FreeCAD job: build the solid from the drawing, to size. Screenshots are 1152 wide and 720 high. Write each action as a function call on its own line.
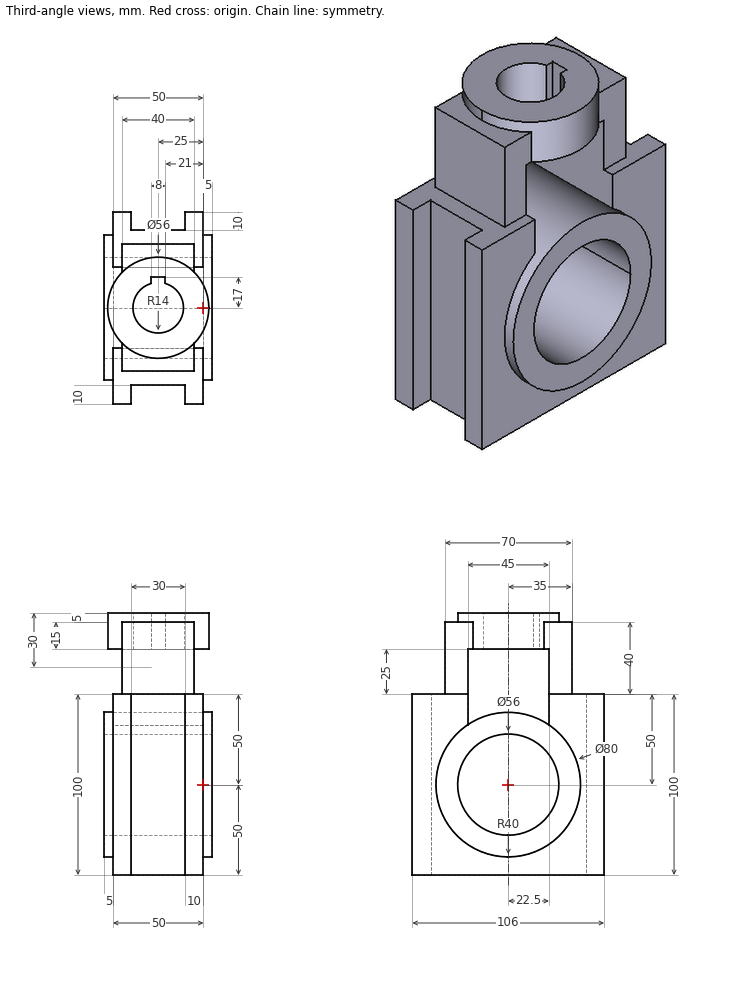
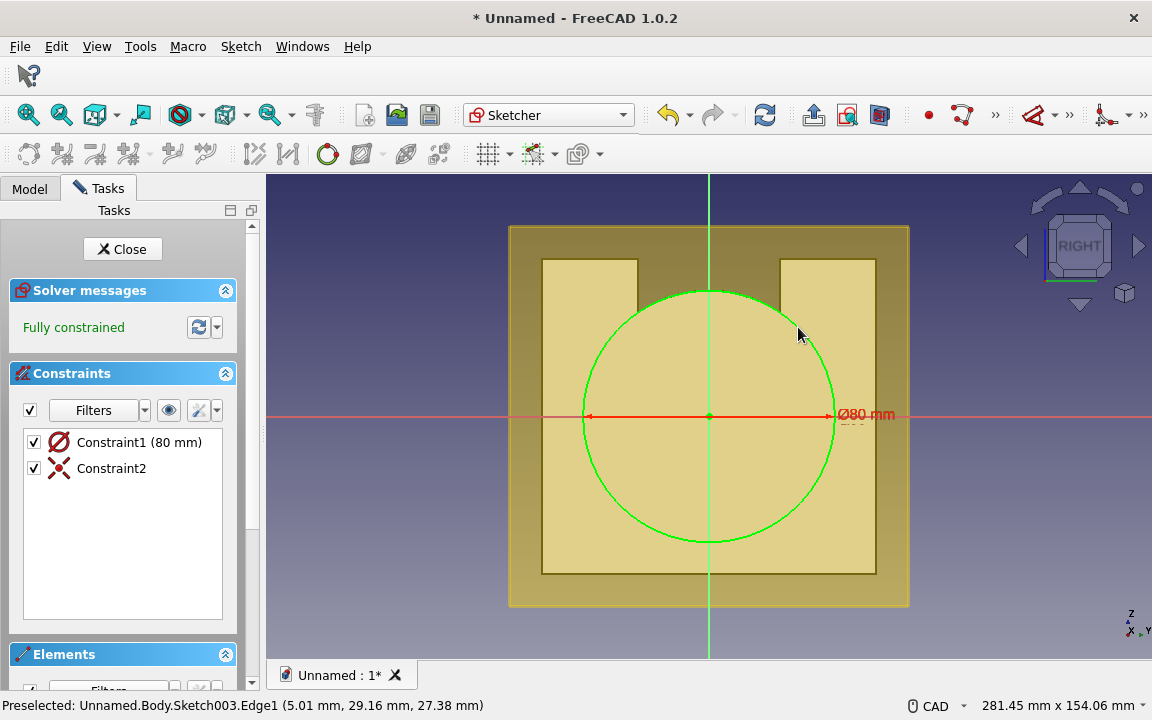
click(123, 249)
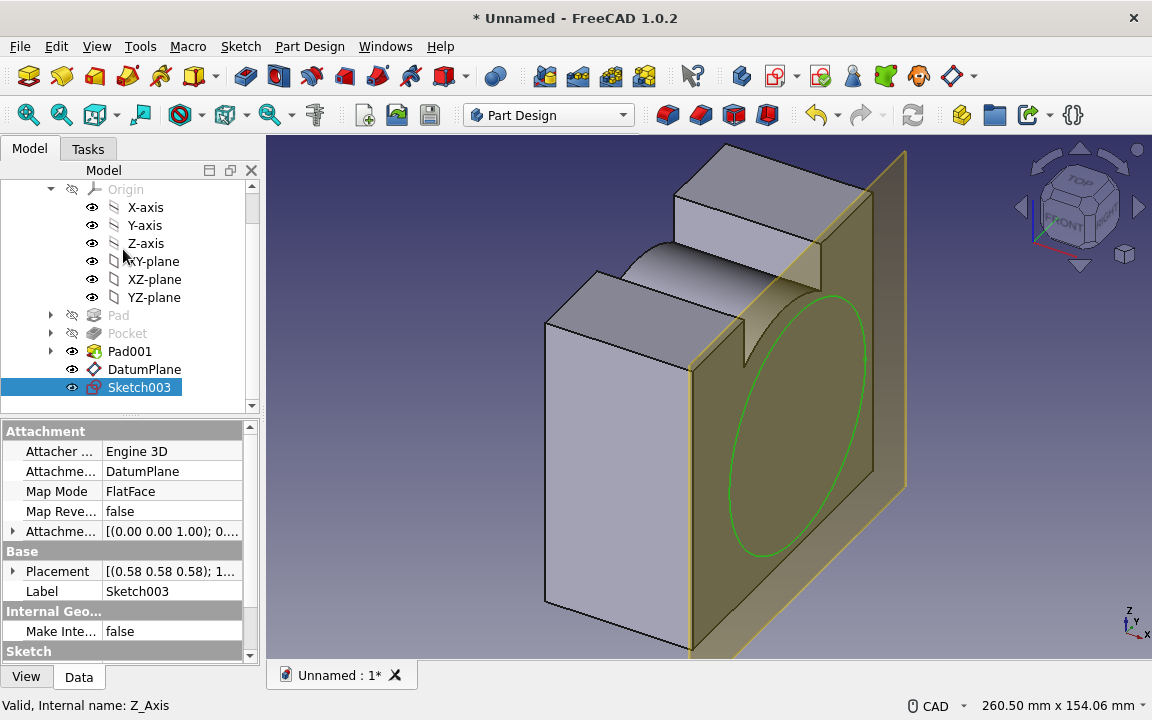
click(29, 76)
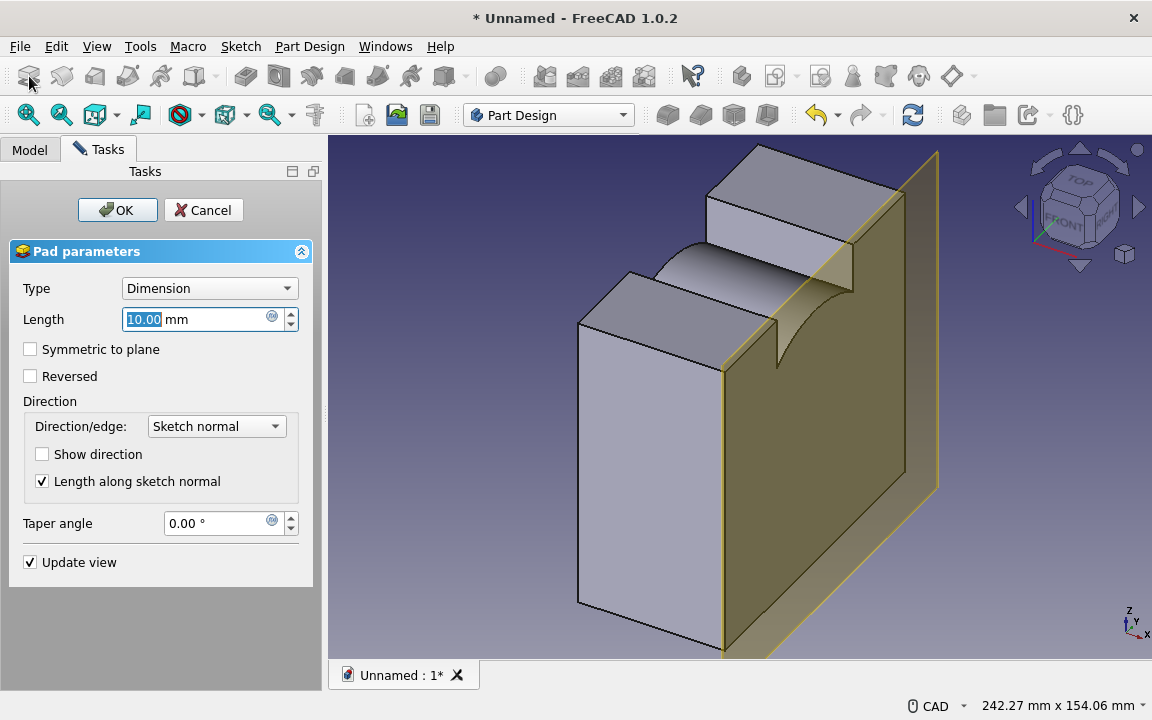
text(5)
key(Tab)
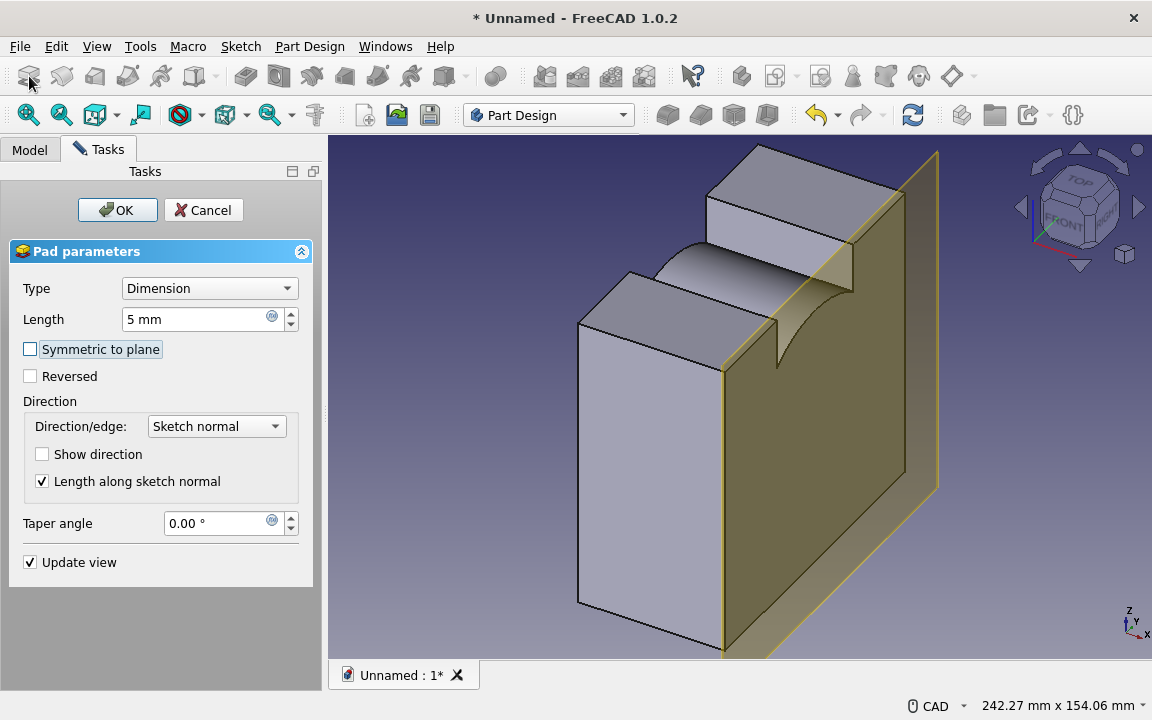
click(31, 376)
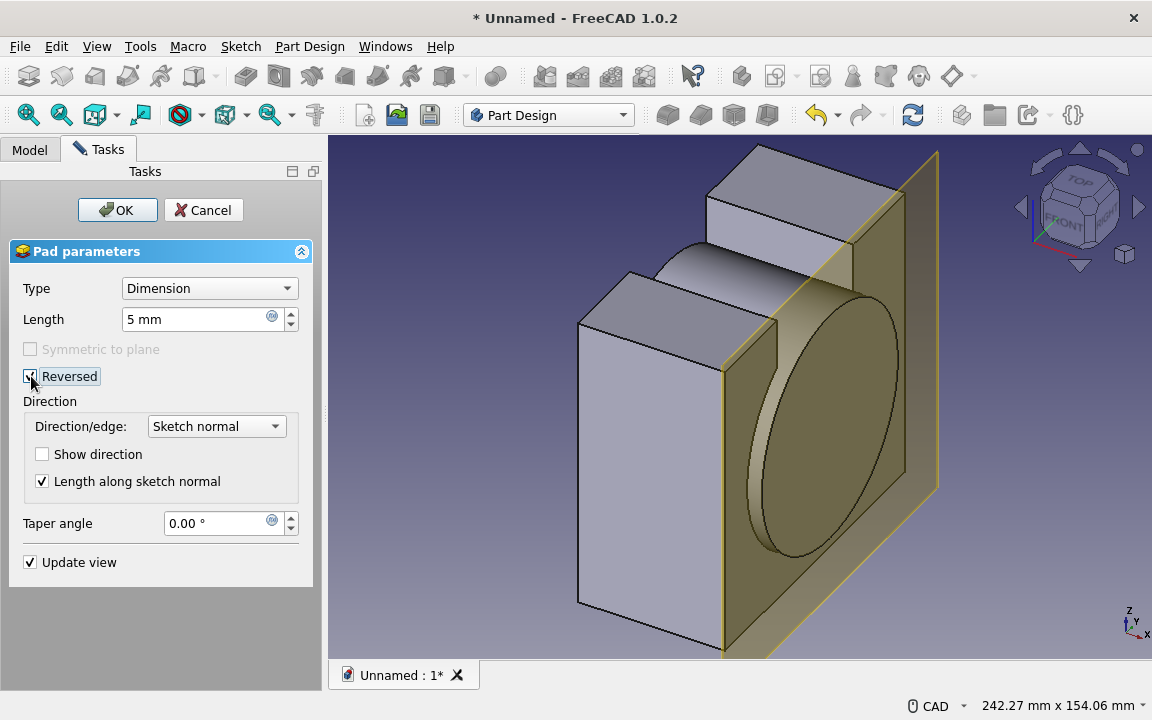
click(118, 210)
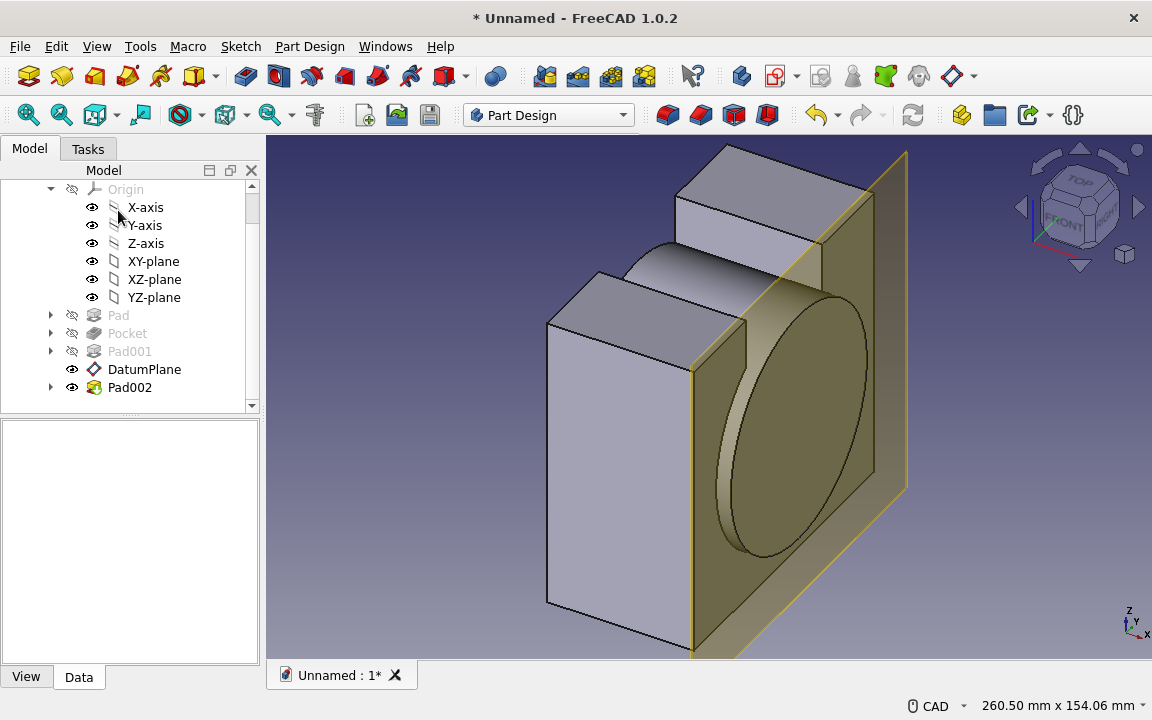
click(117, 369)
key(space)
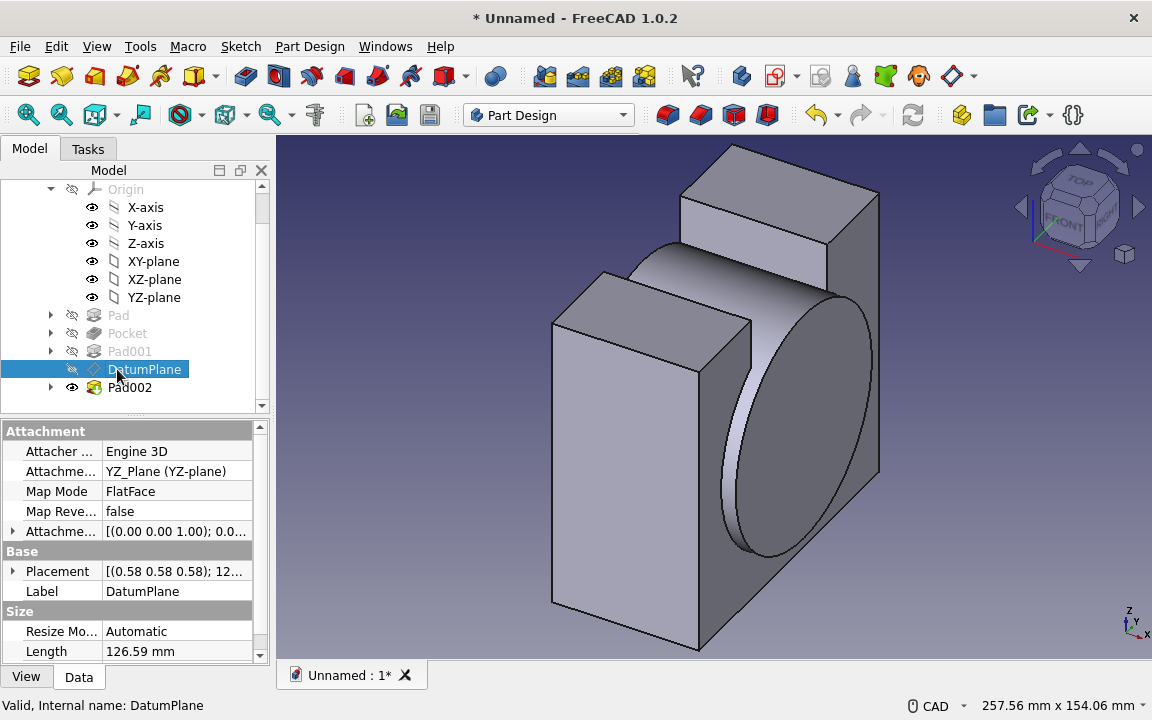
click(804, 426)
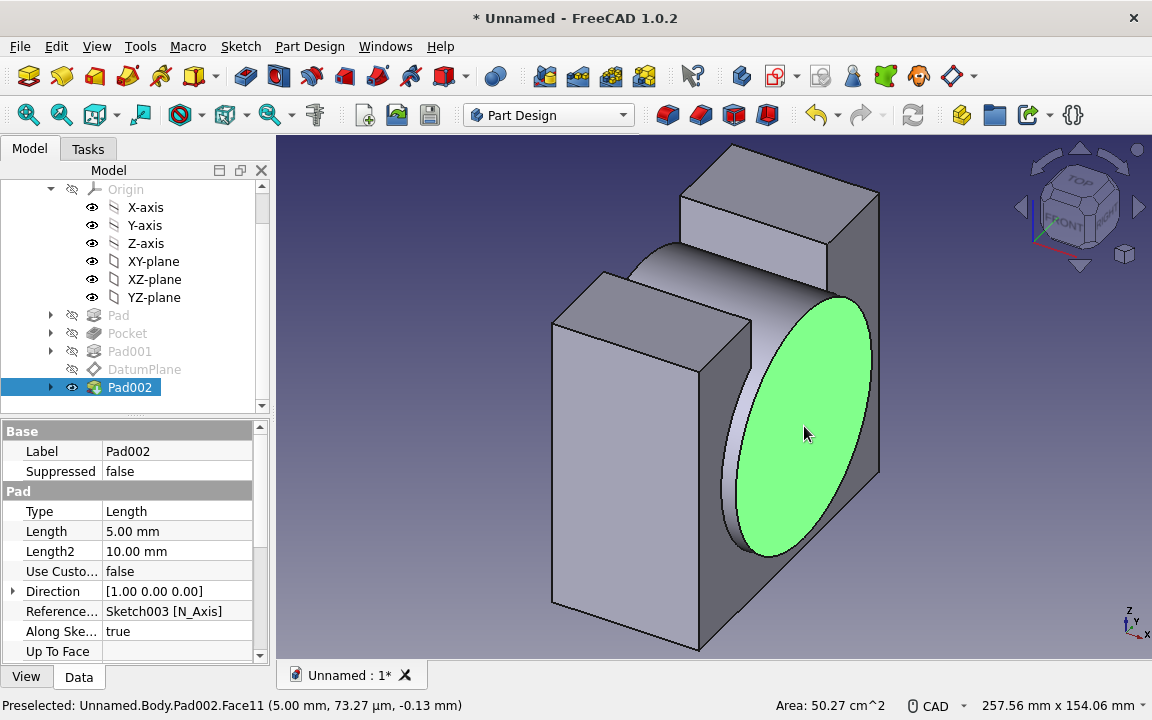
click(774, 76)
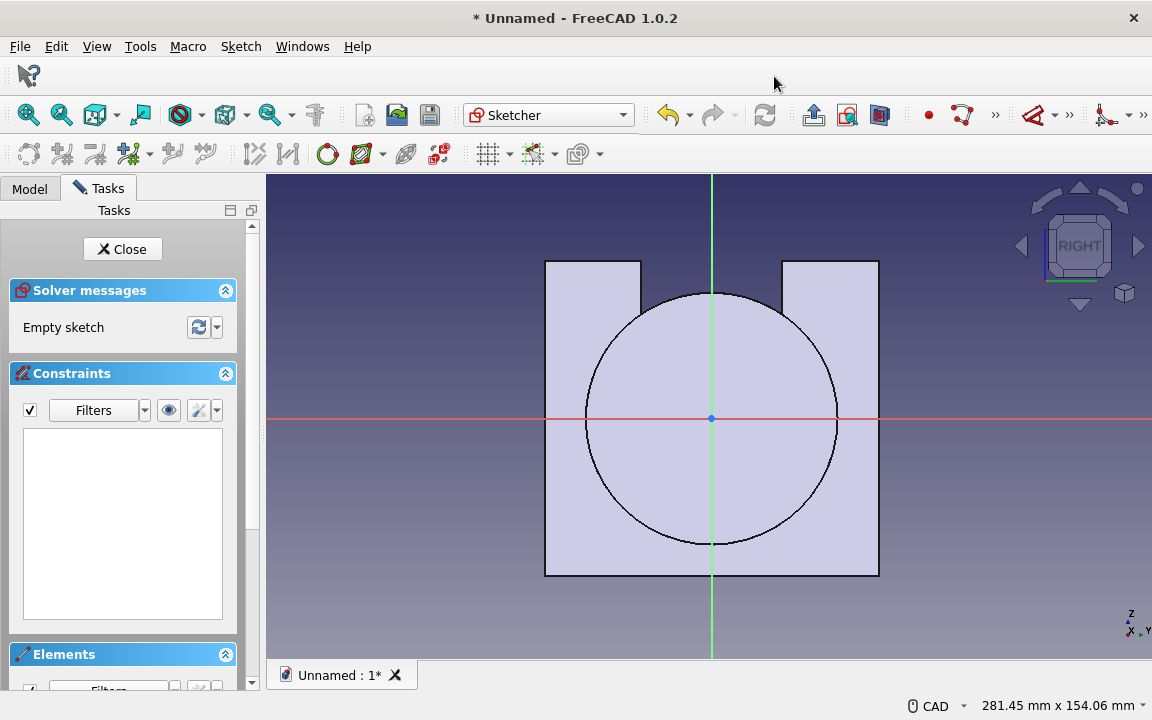
scroll(798, 421, up, 3)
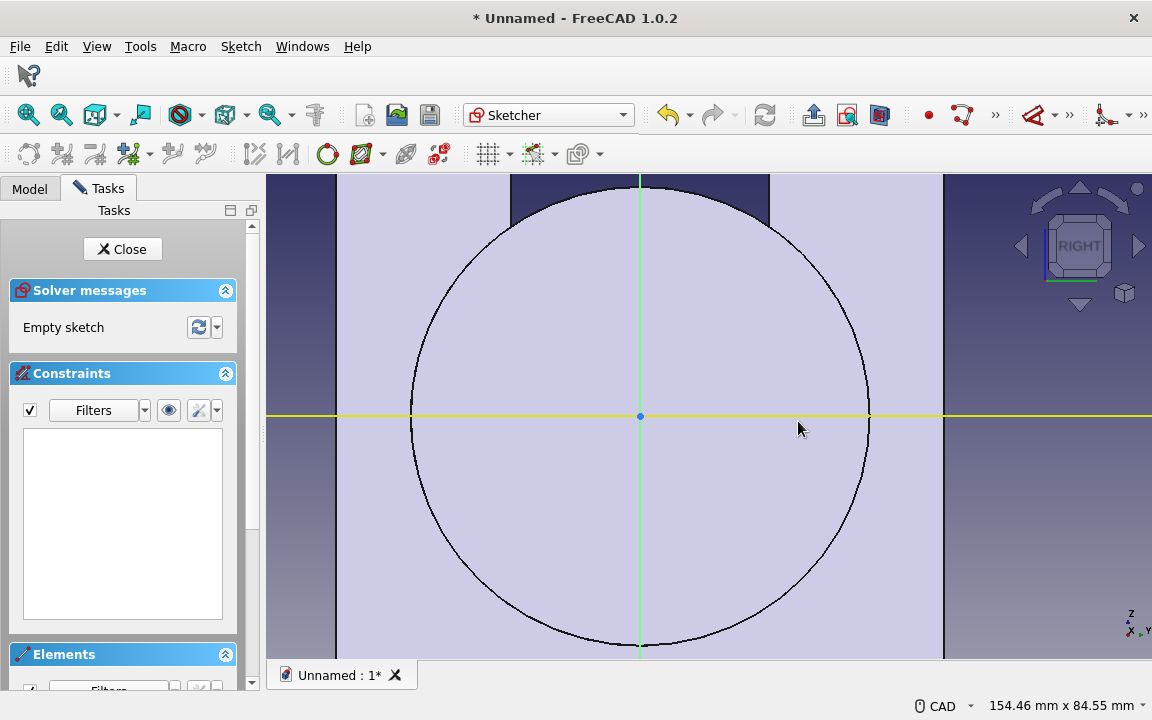
key(g)
key(c)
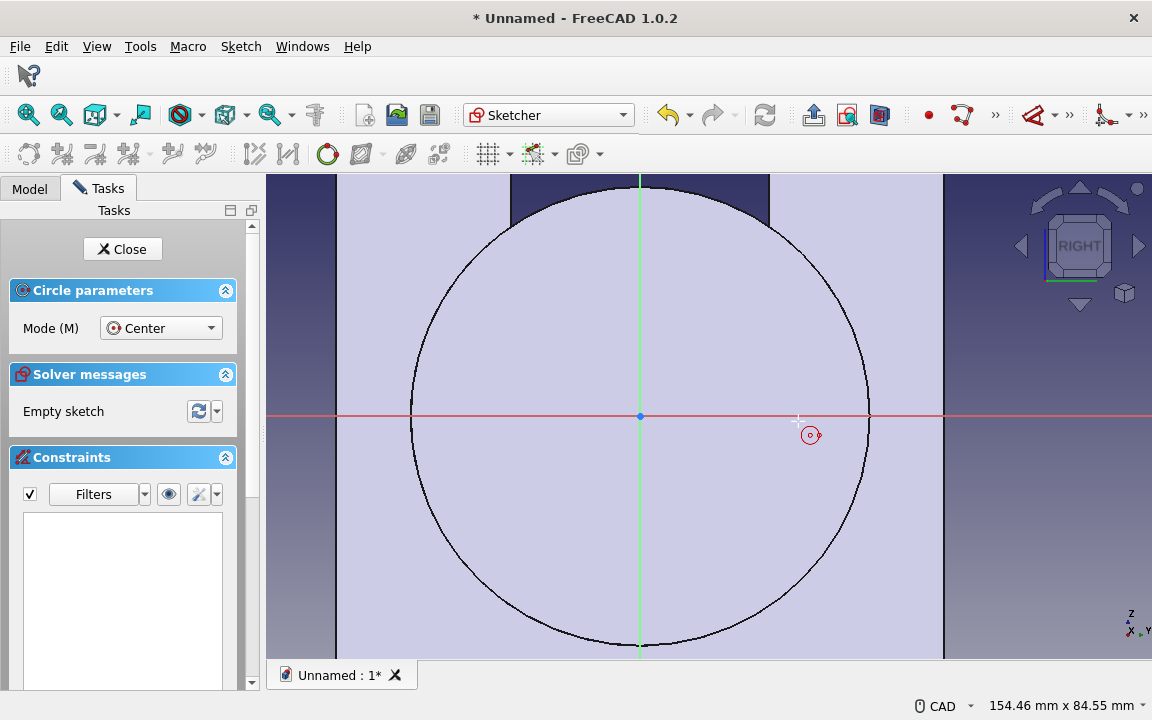
click(640, 416)
move(754, 303)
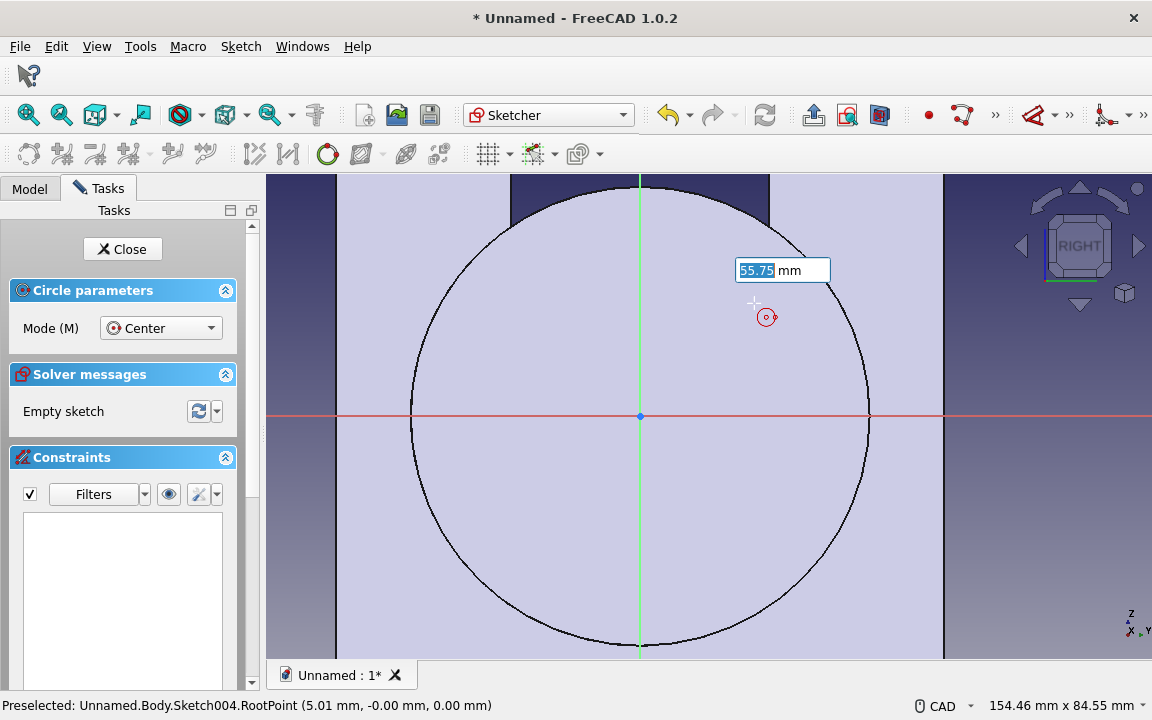
text(56)
key(Return)
key(Escape)